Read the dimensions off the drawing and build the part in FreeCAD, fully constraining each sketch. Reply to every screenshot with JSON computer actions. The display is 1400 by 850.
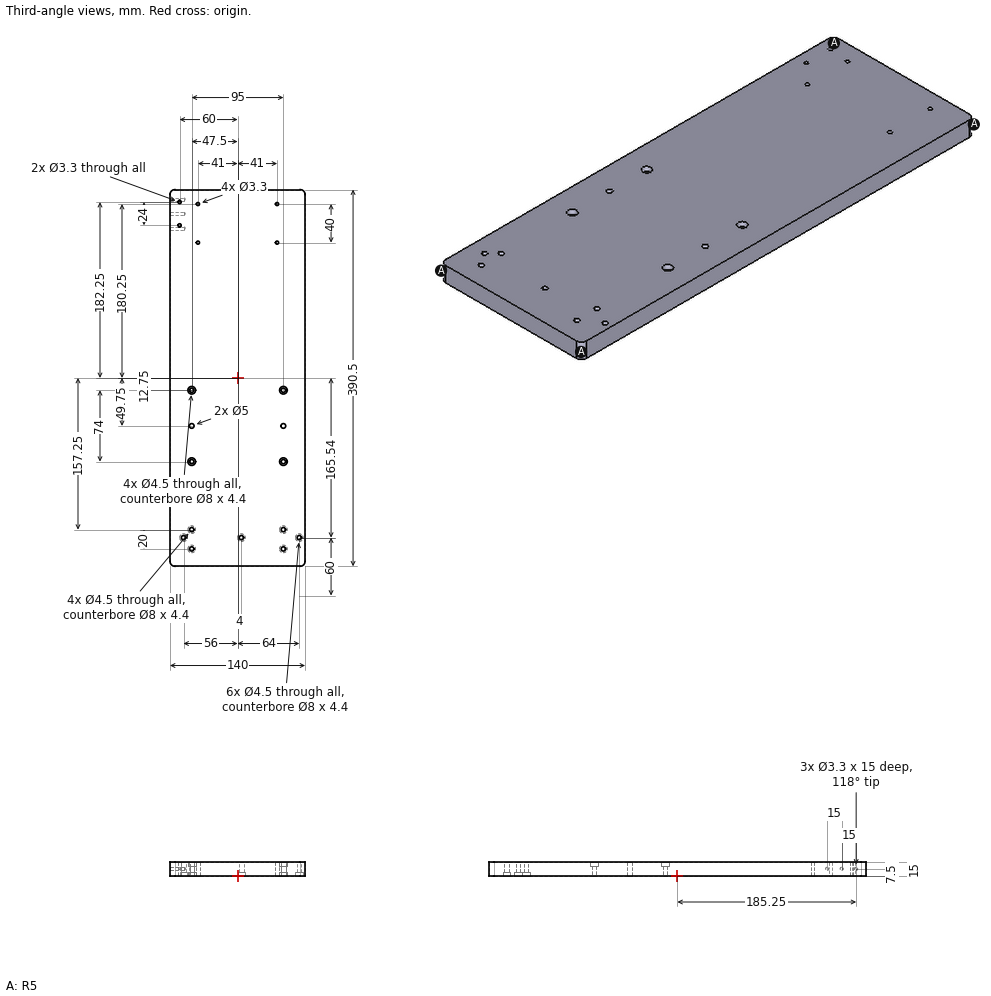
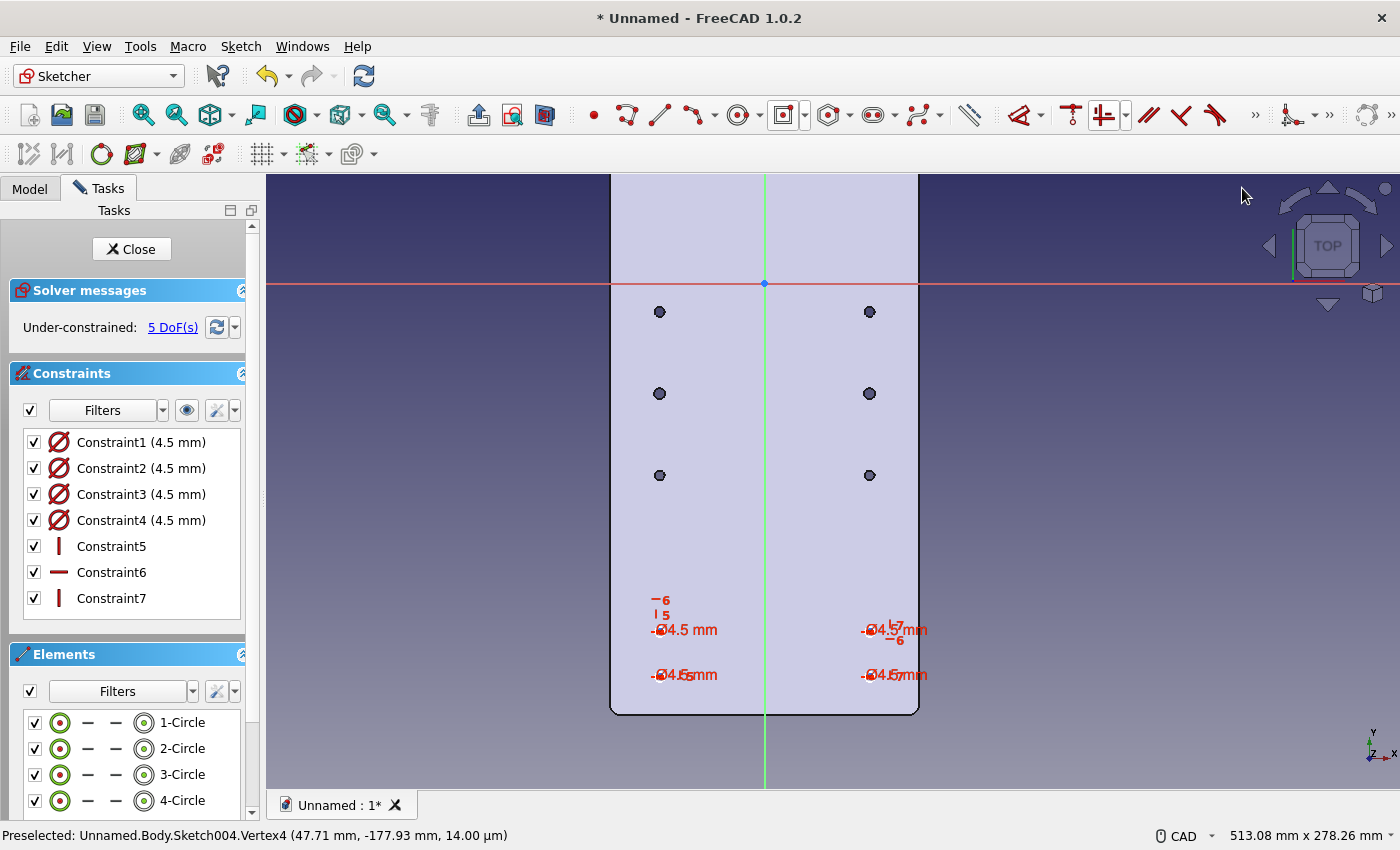
{"action": "left_click", "coordinate": [660, 677]}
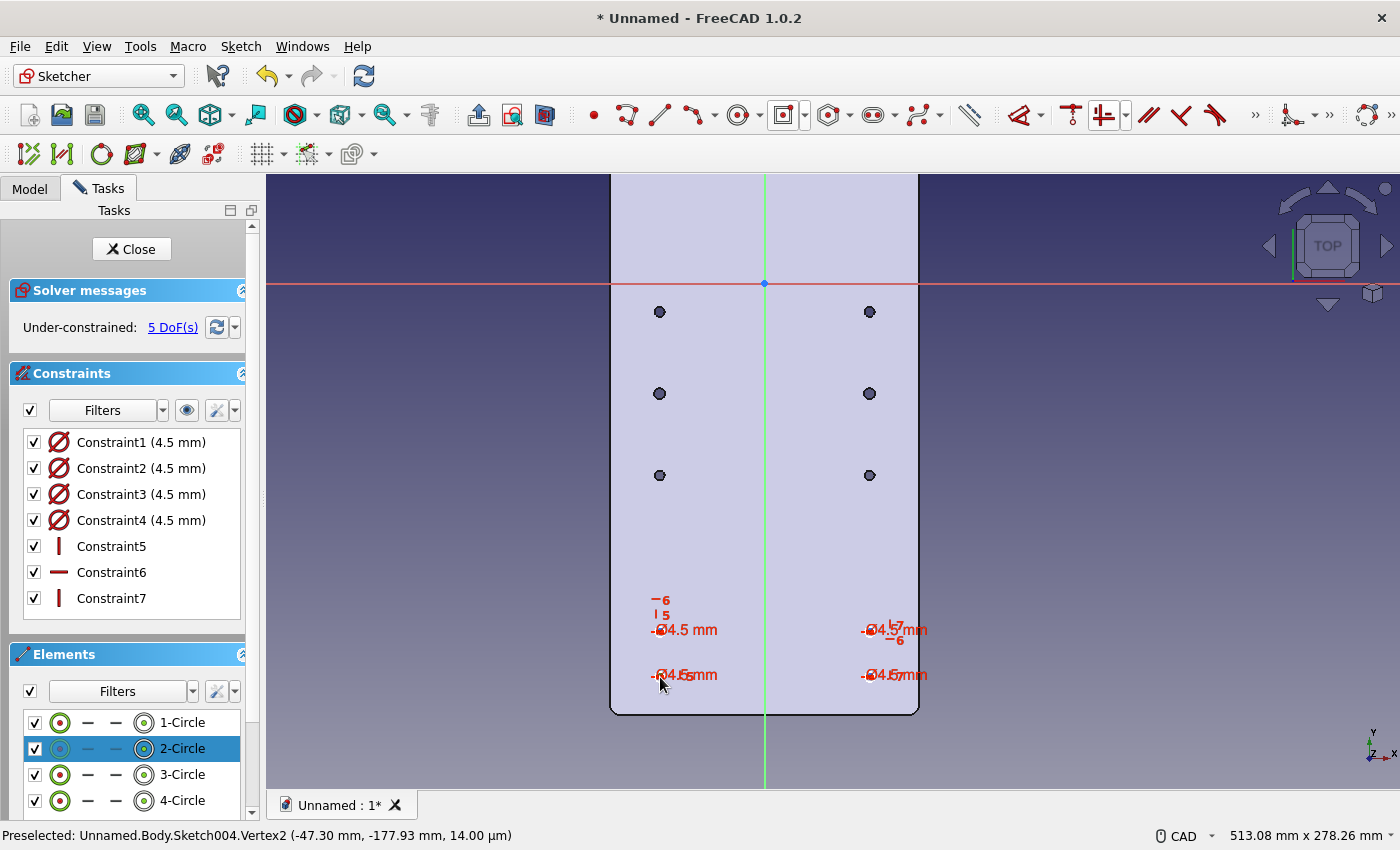
{"action": "left_click", "coordinate": [870, 677]}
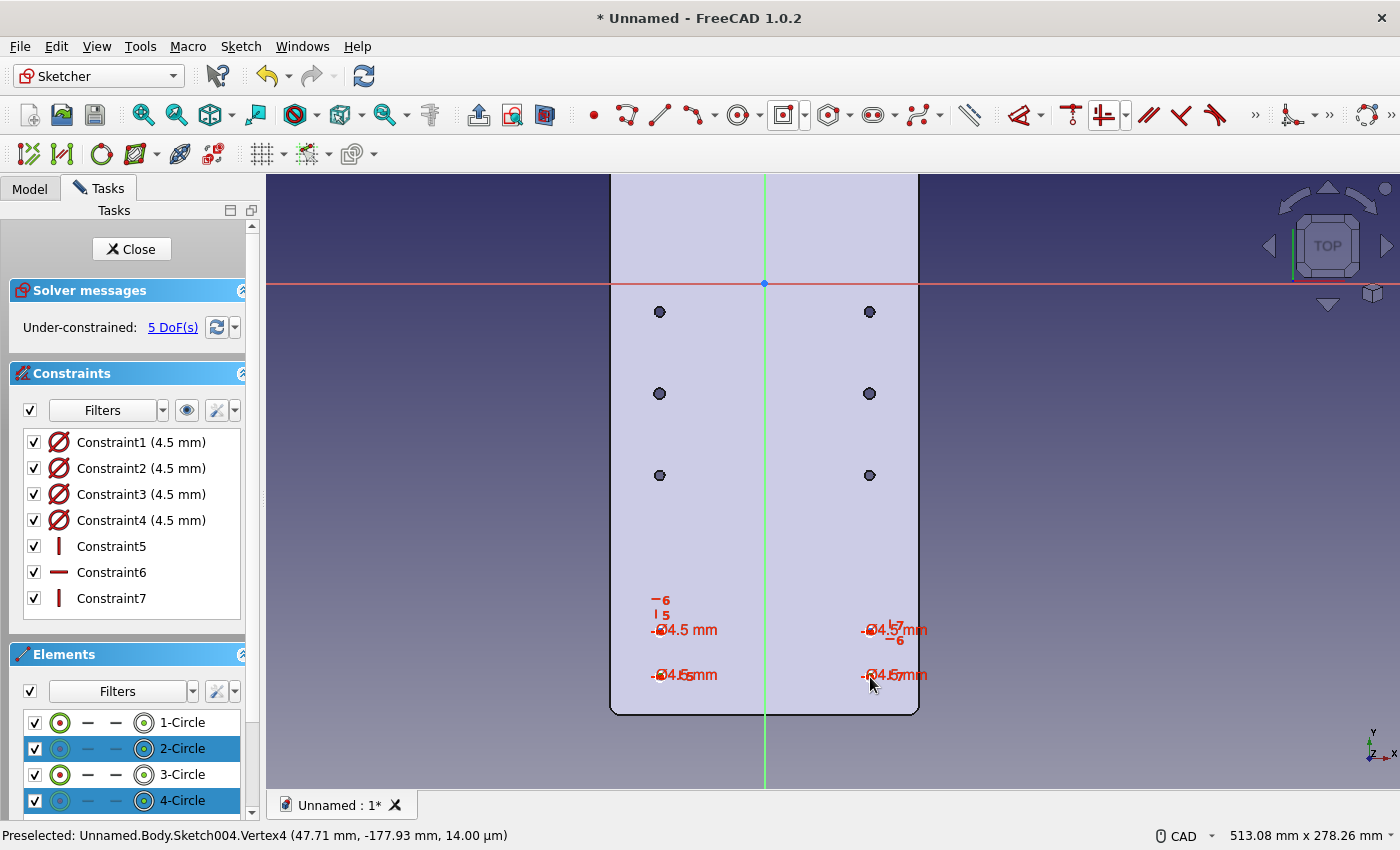
{"action": "key", "text": "h"}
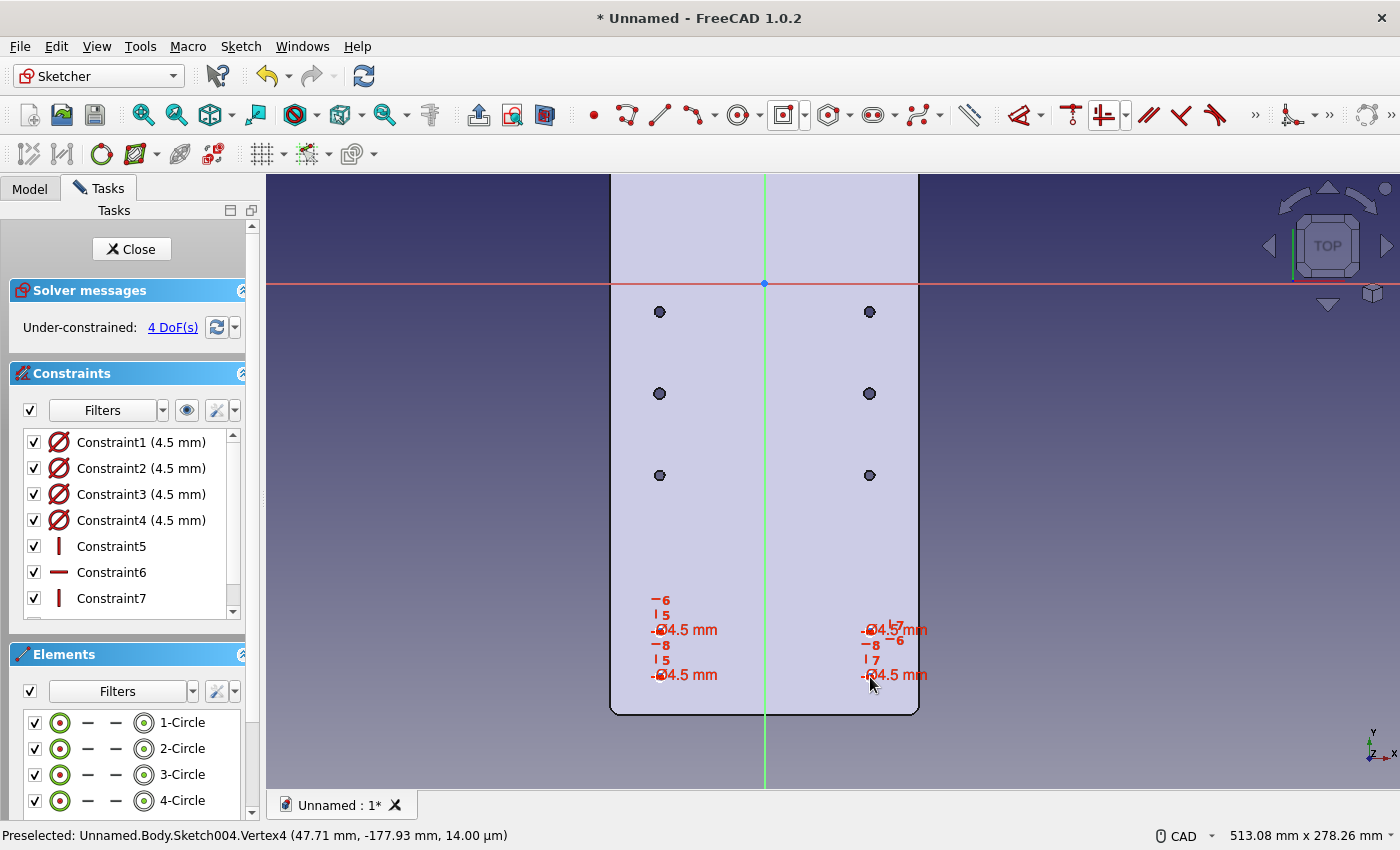
{"action": "left_click", "coordinate": [1018, 116]}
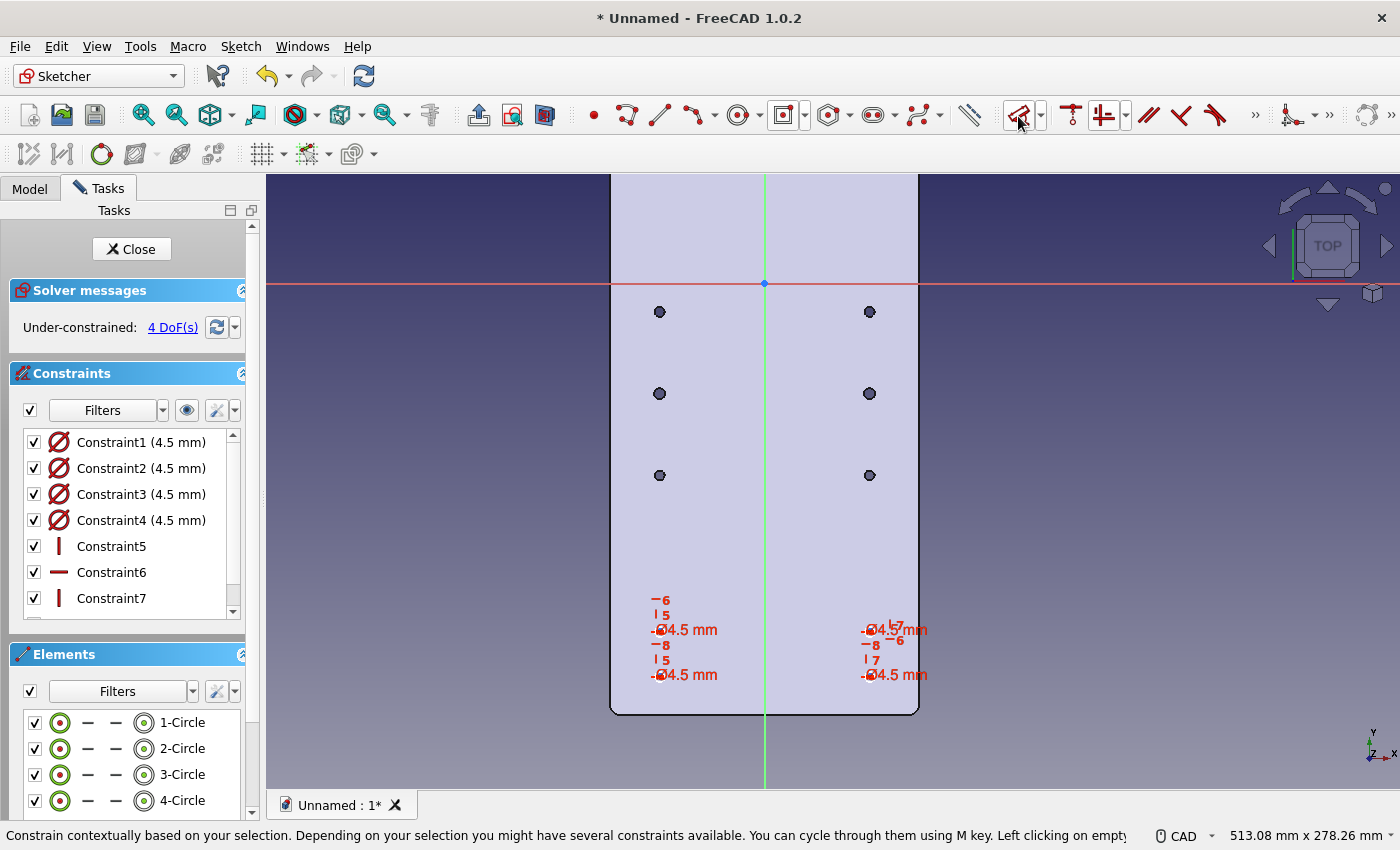
{"action": "left_click", "coordinate": [660, 632]}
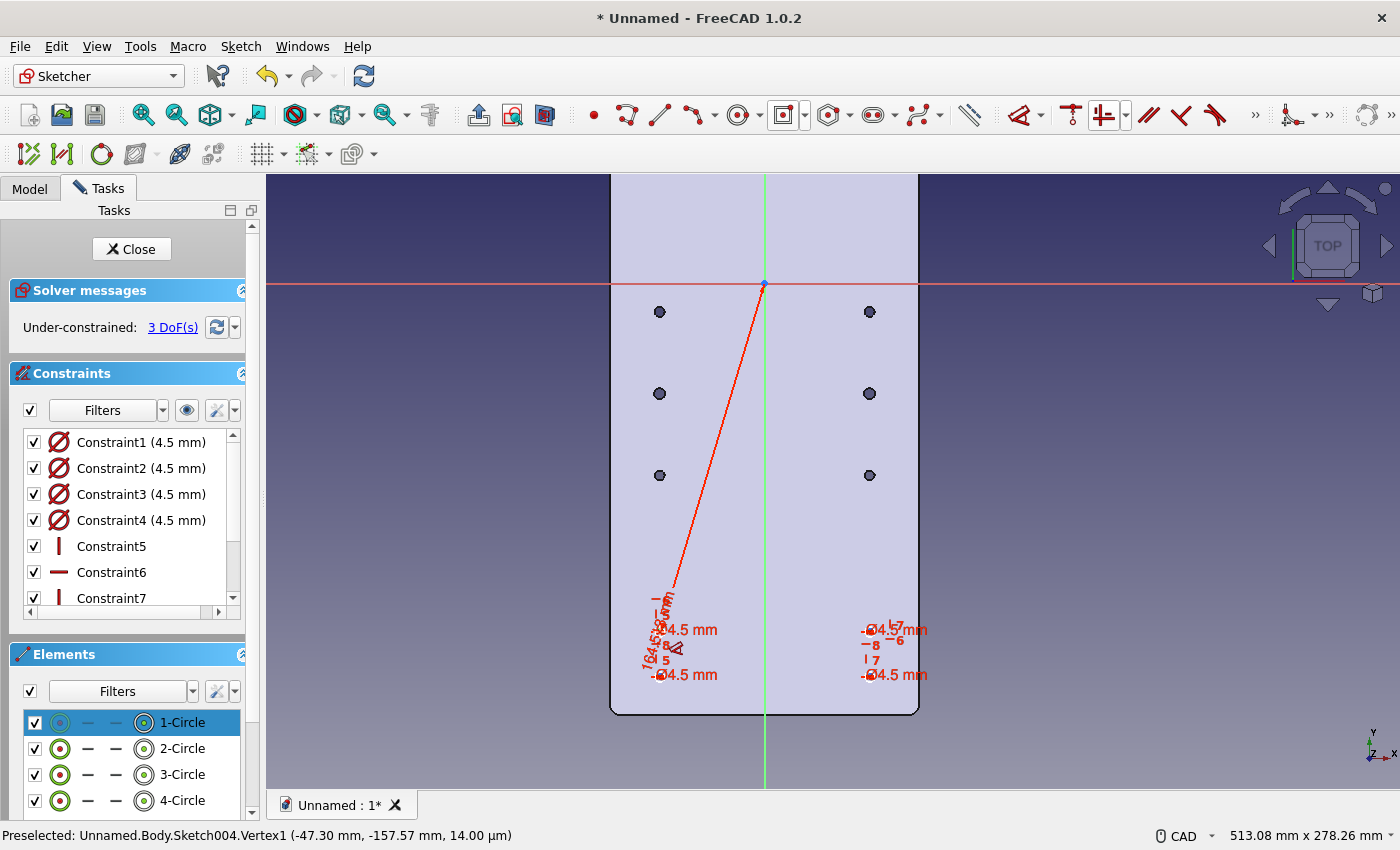
{"action": "left_click", "coordinate": [660, 677]}
{"action": "left_click", "coordinate": [626, 655]}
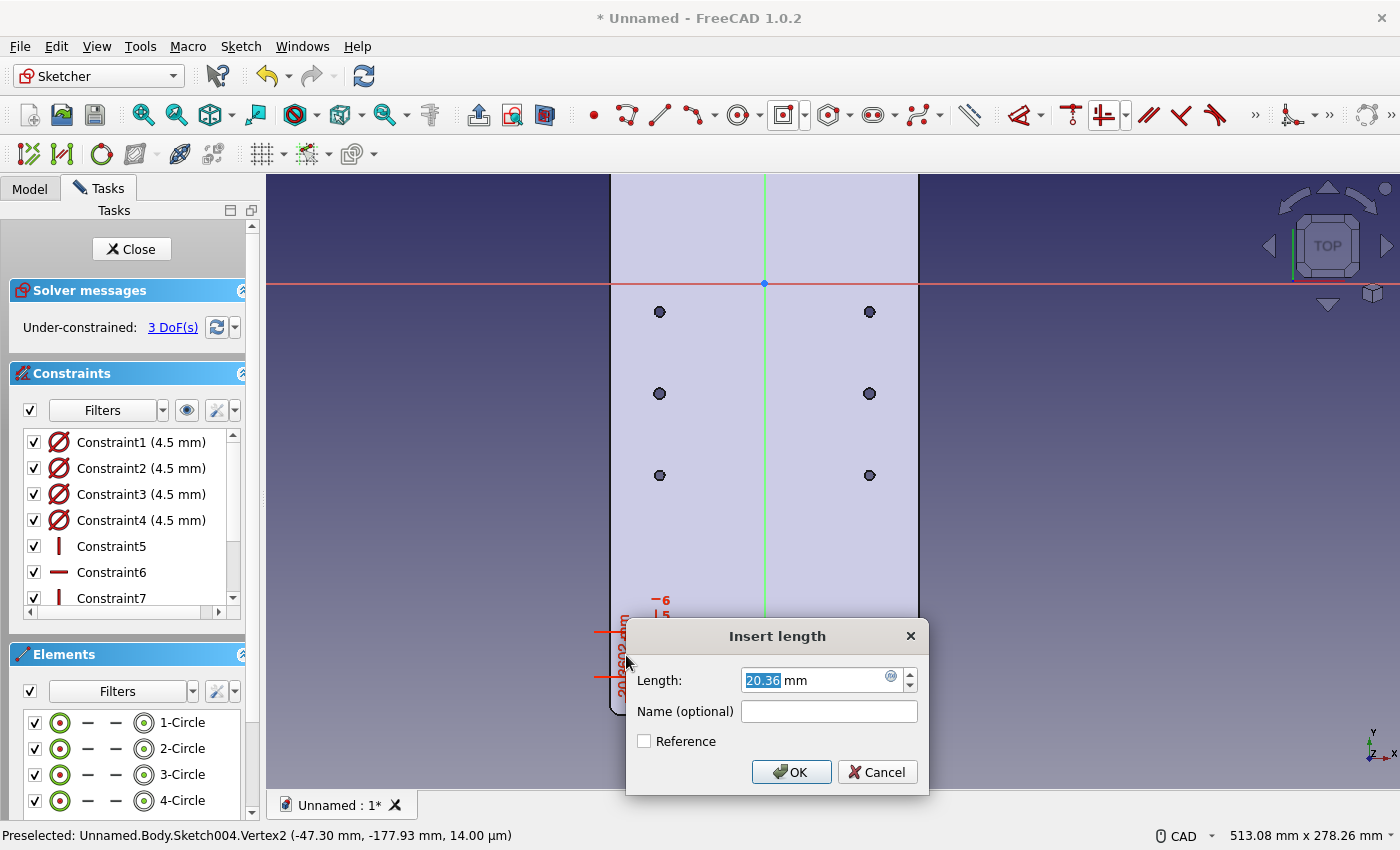
{"action": "type", "text": "20"}
{"action": "key", "text": "Return"}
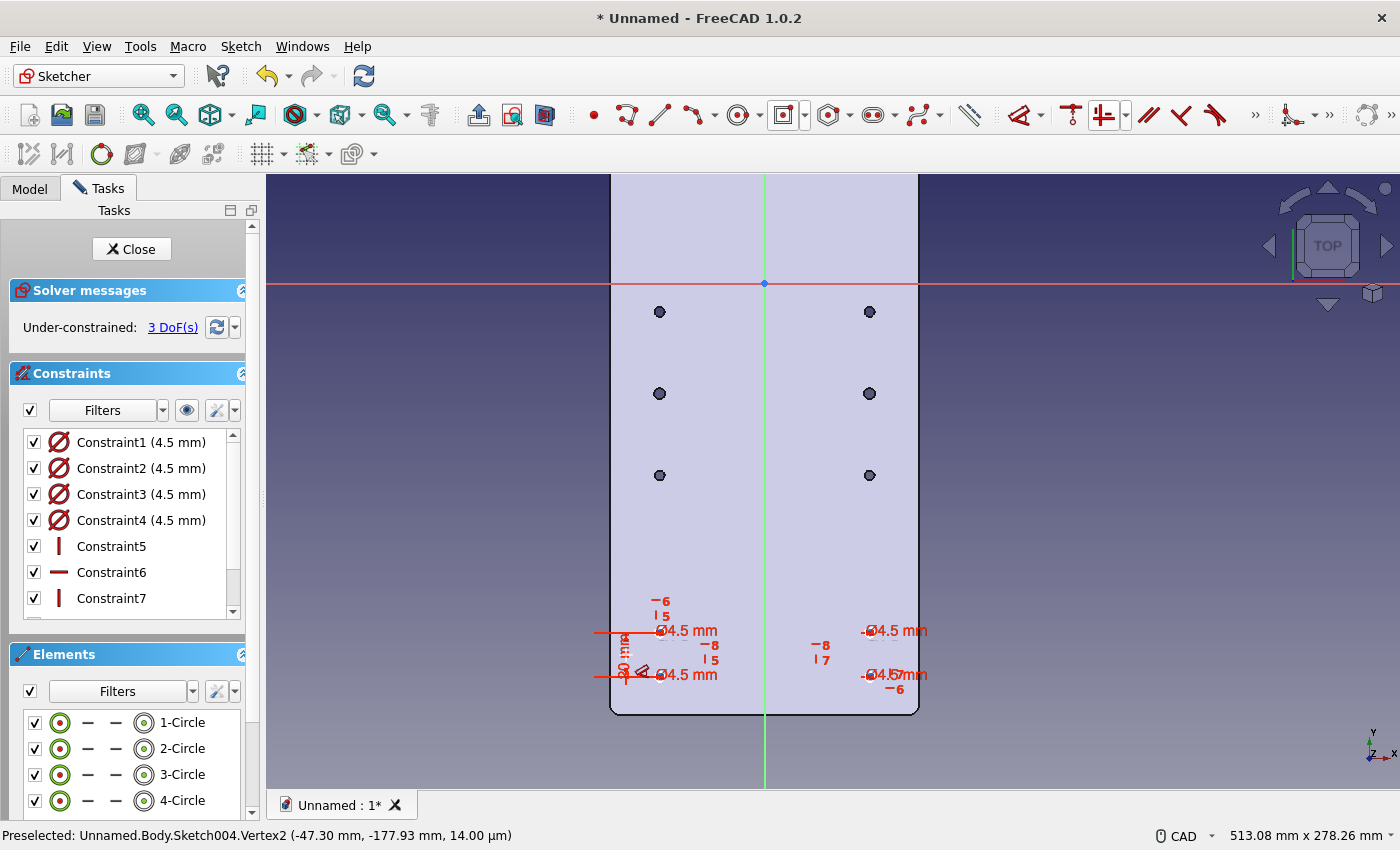
{"action": "left_click", "coordinate": [660, 633]}